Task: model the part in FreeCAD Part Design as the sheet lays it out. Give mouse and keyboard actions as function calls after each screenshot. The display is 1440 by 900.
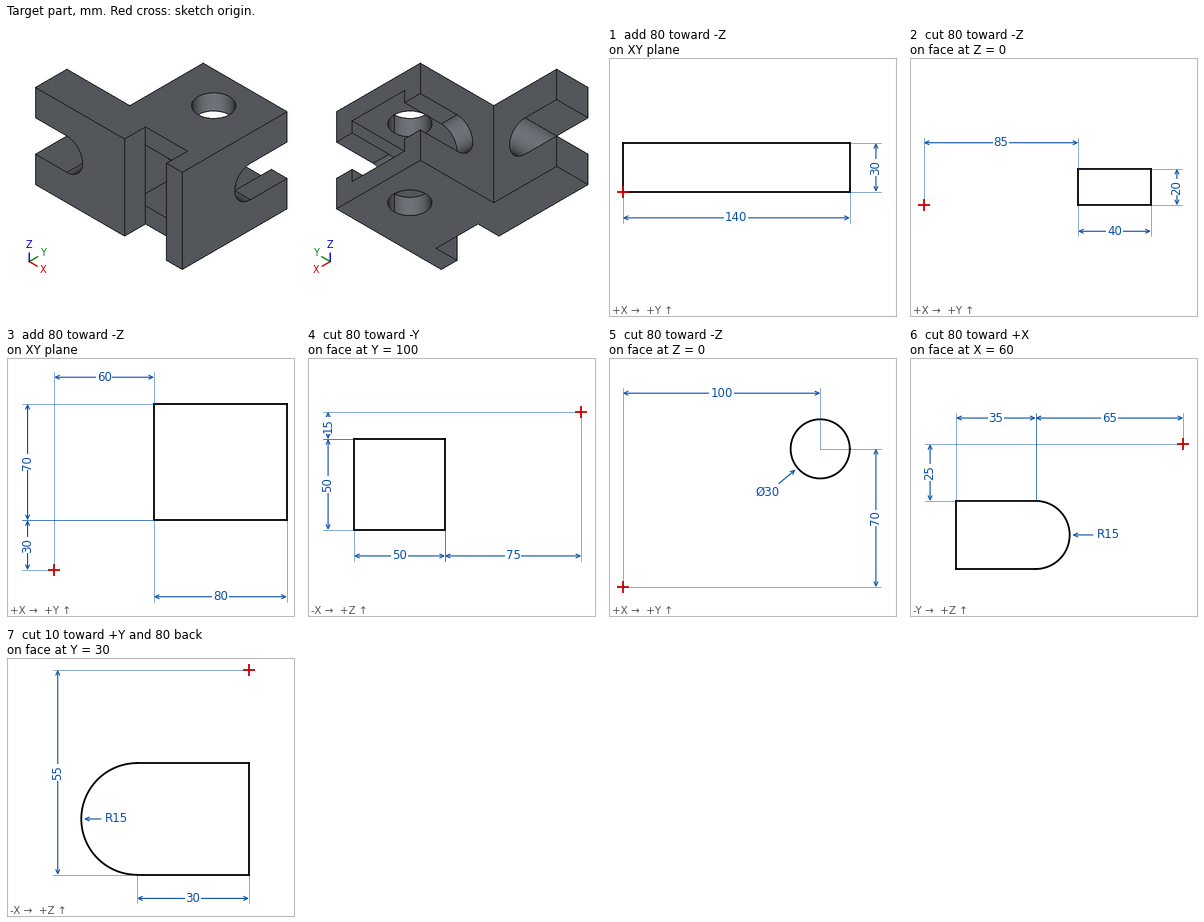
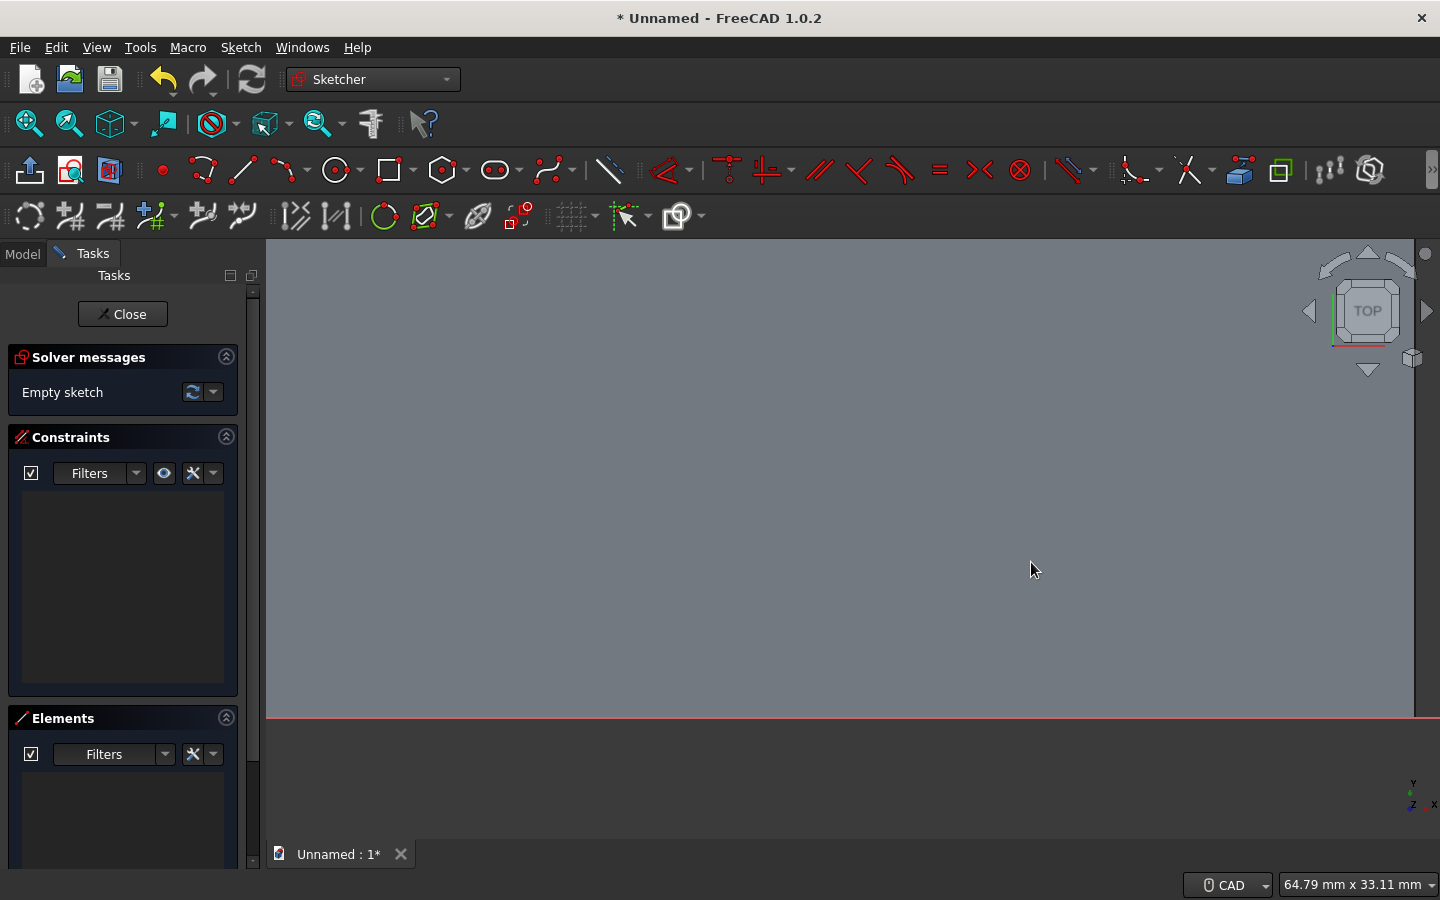
key(g)
key(r)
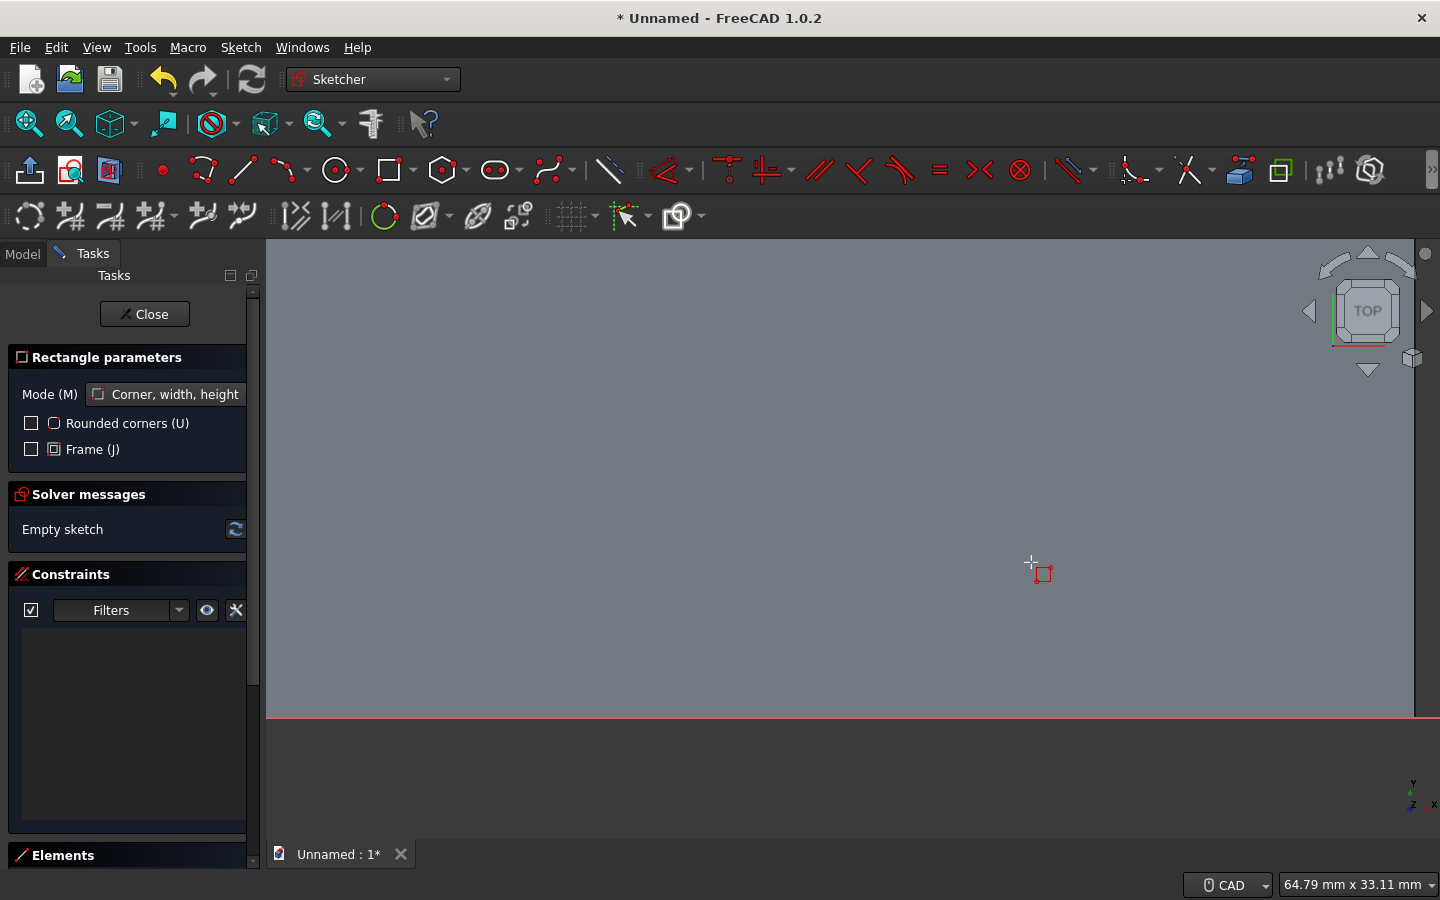
click(419, 355)
click(1143, 718)
key(Escape)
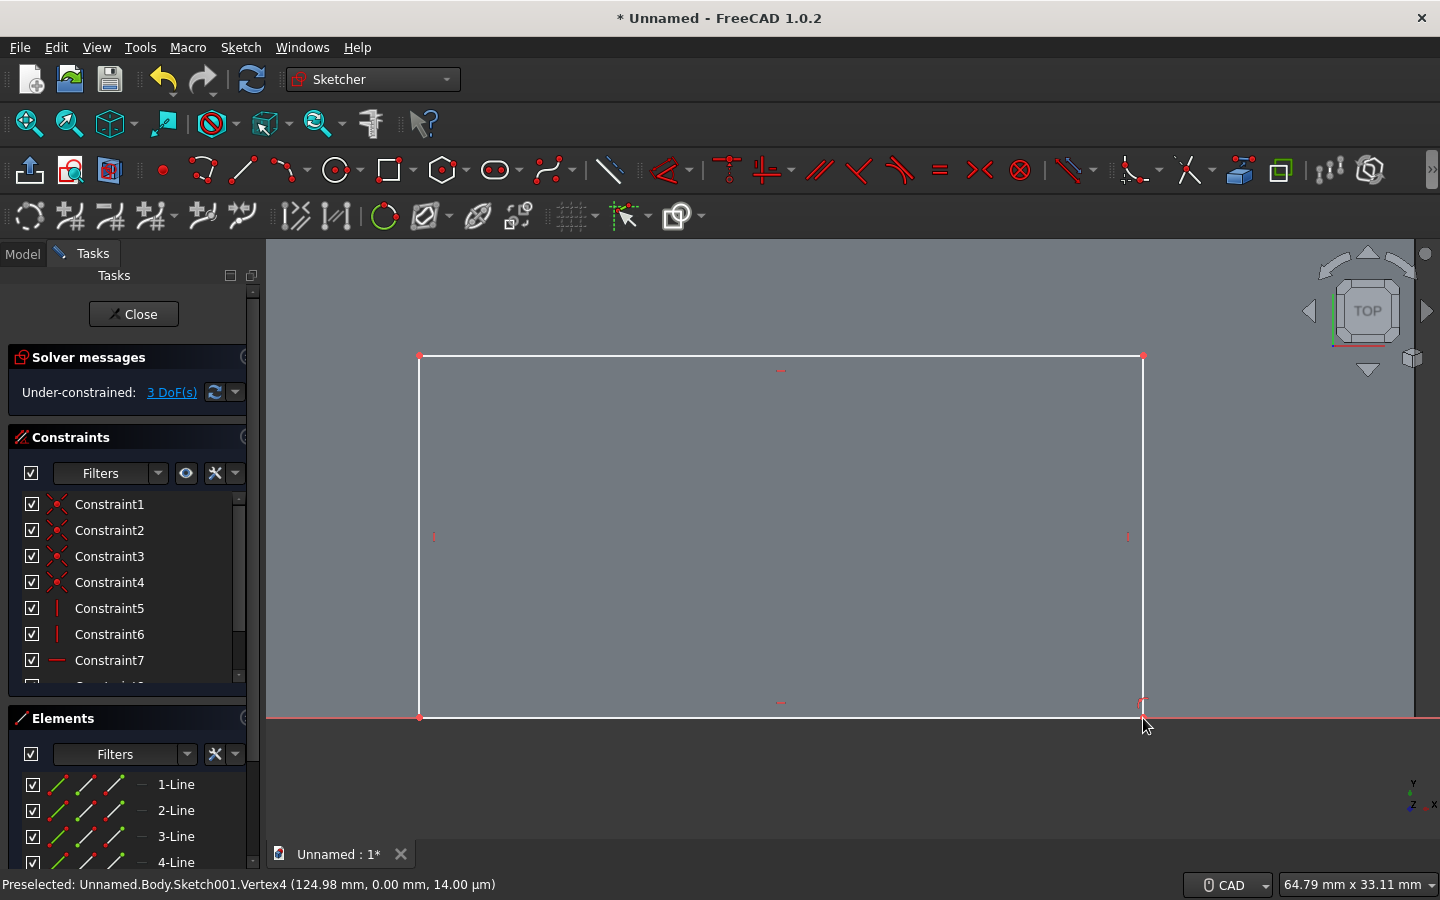
click(664, 170)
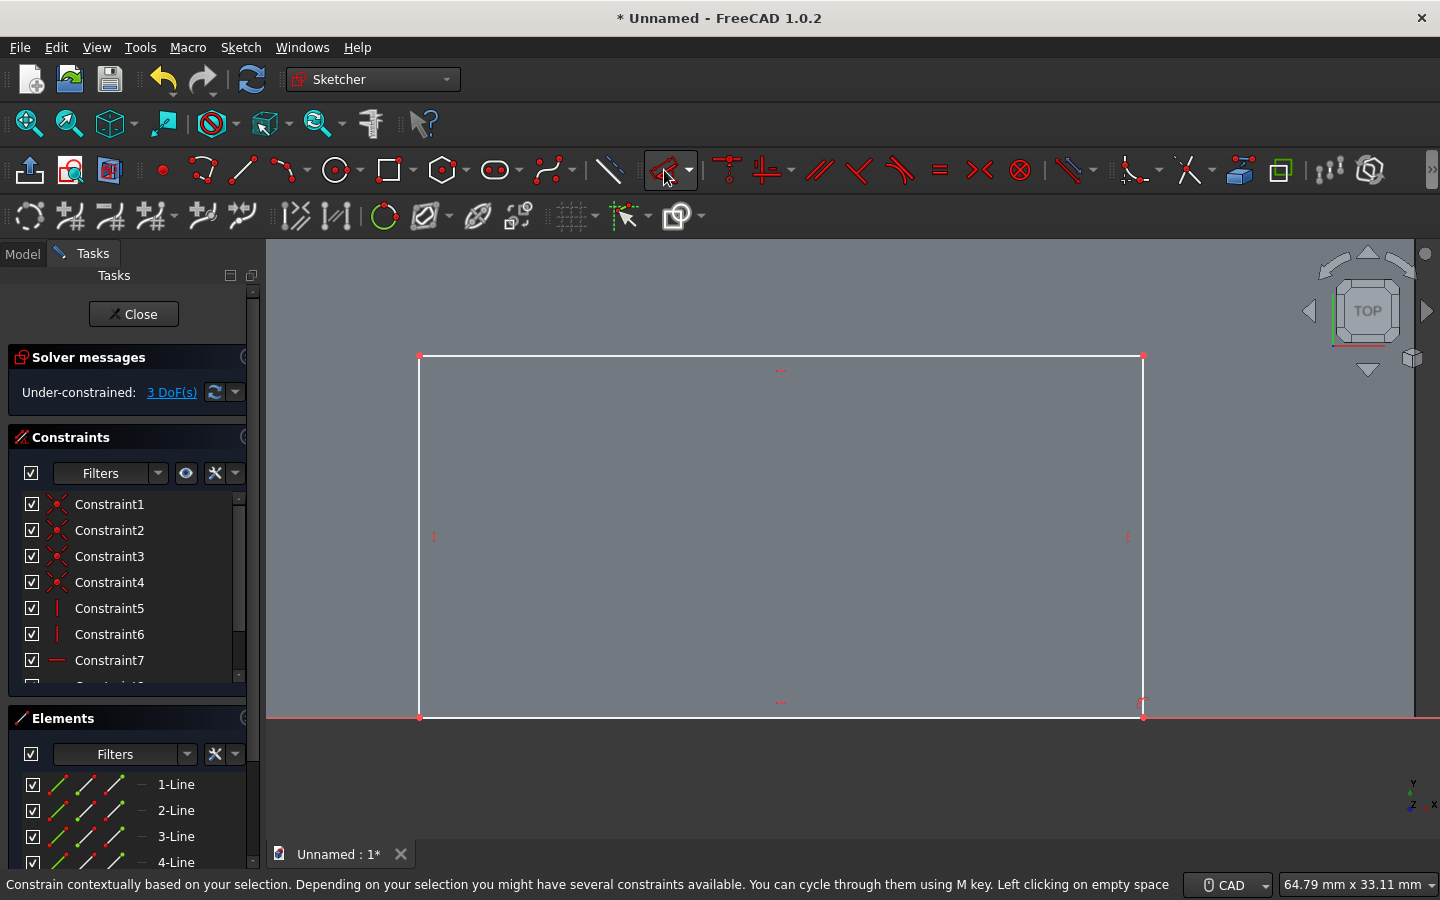
click(419, 465)
click(385, 537)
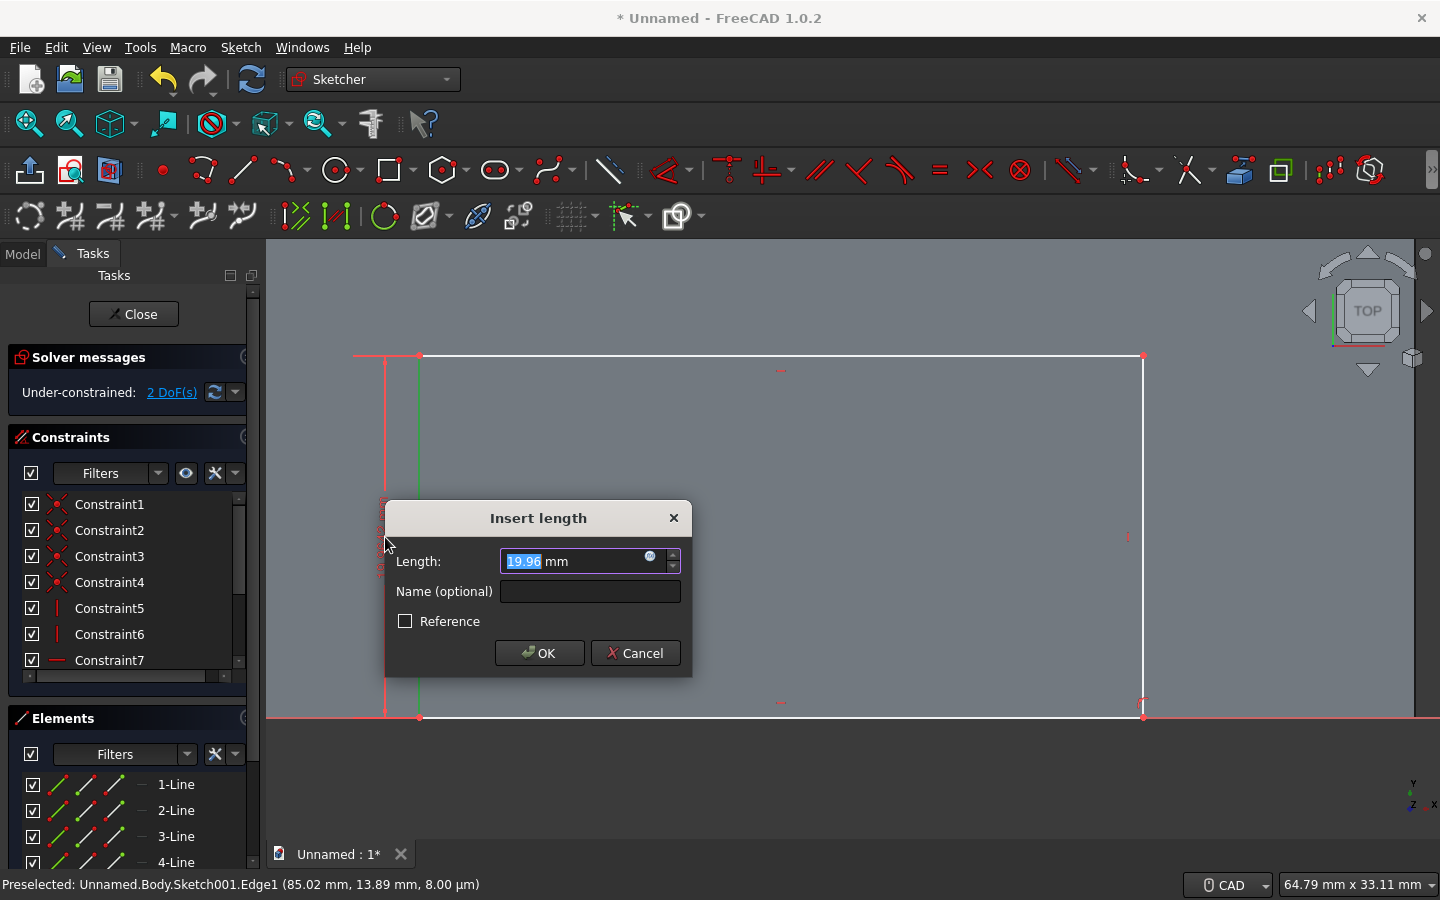
text(20)
key(Return)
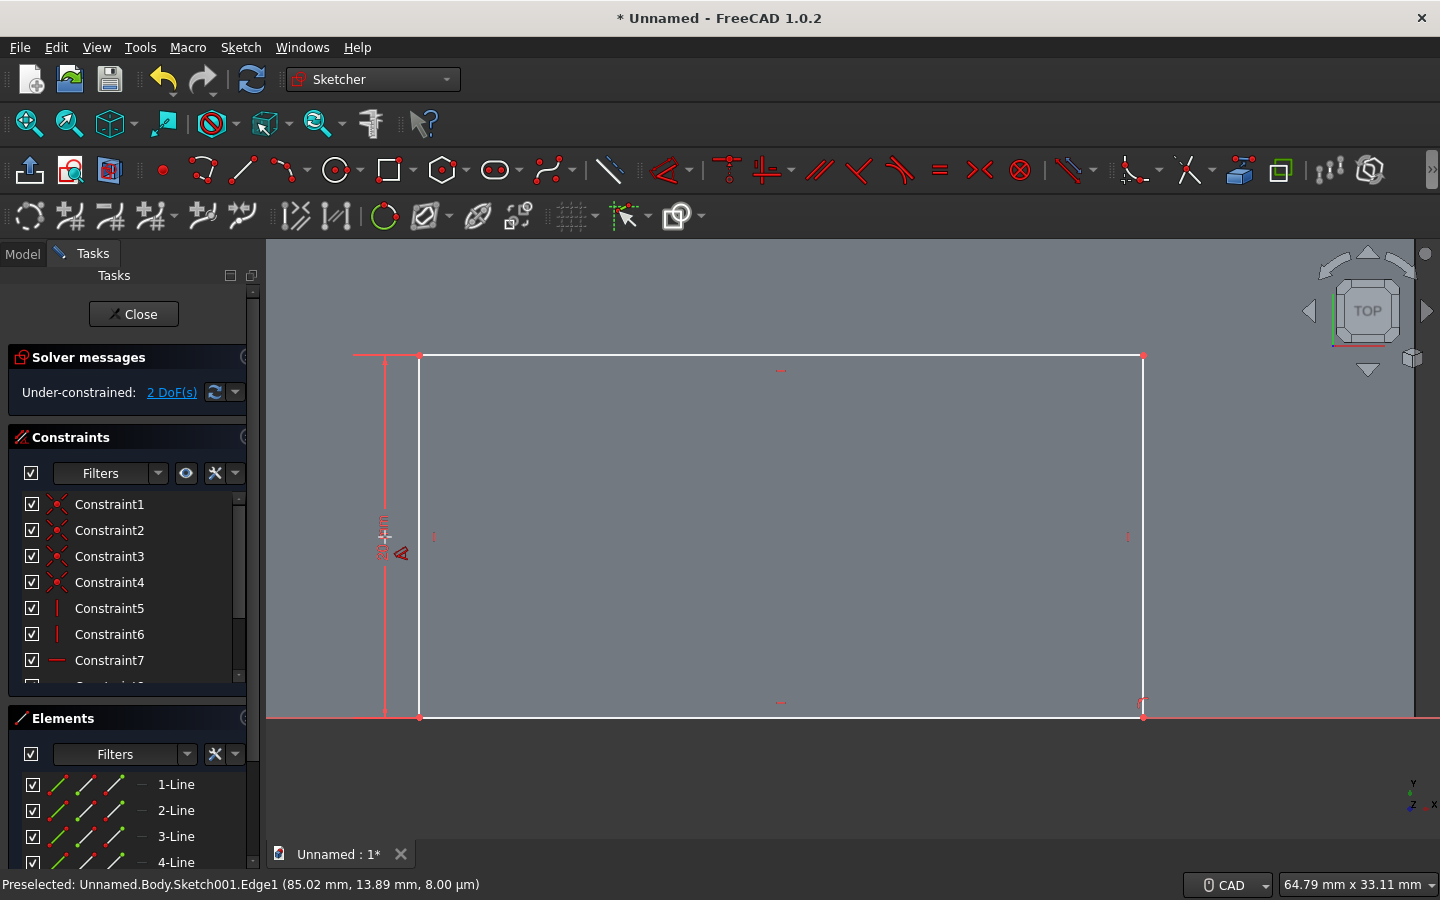
click(636, 718)
click(781, 752)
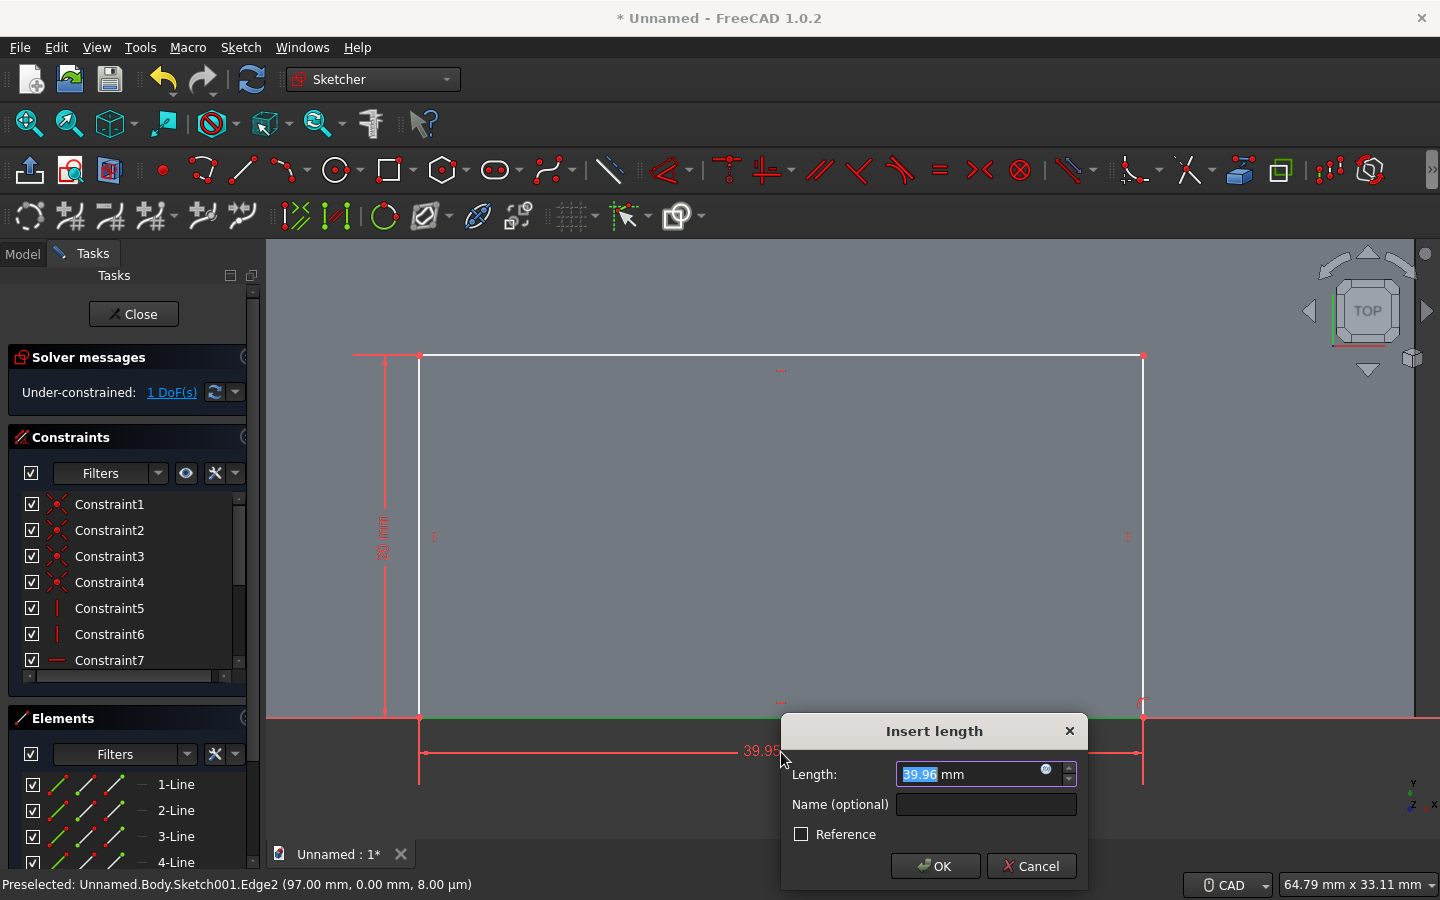
text(40)
key(Return)